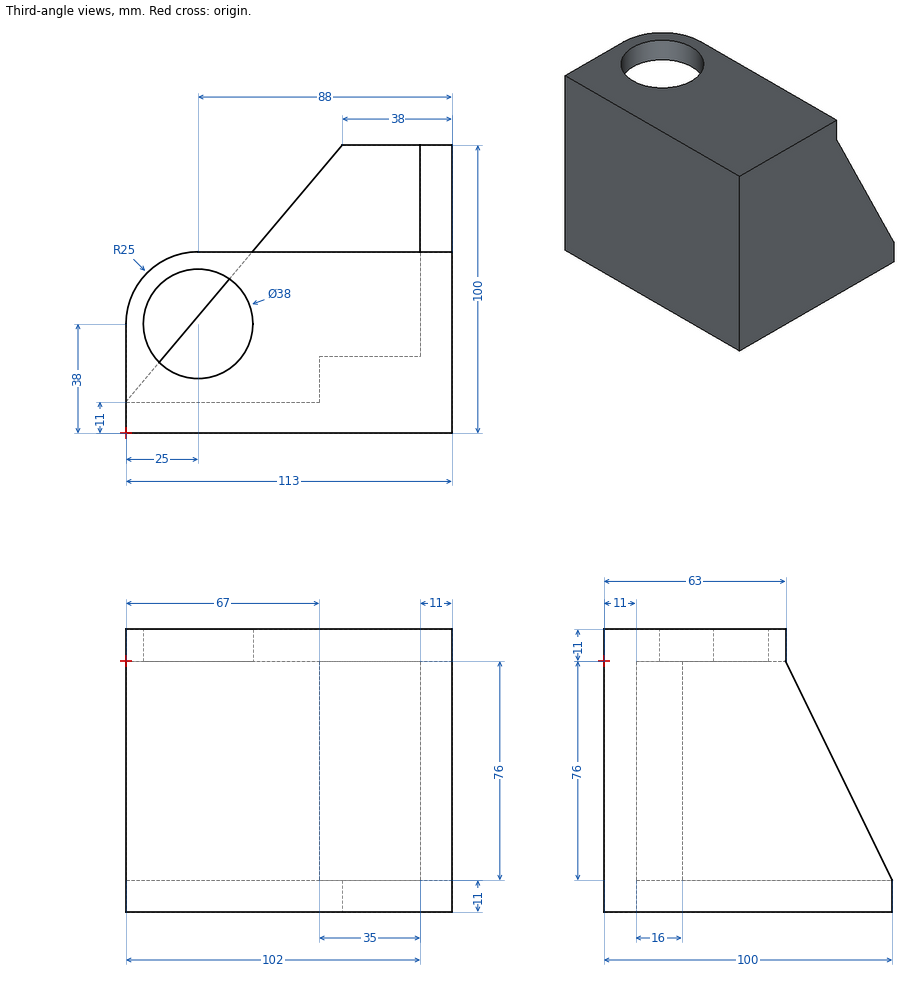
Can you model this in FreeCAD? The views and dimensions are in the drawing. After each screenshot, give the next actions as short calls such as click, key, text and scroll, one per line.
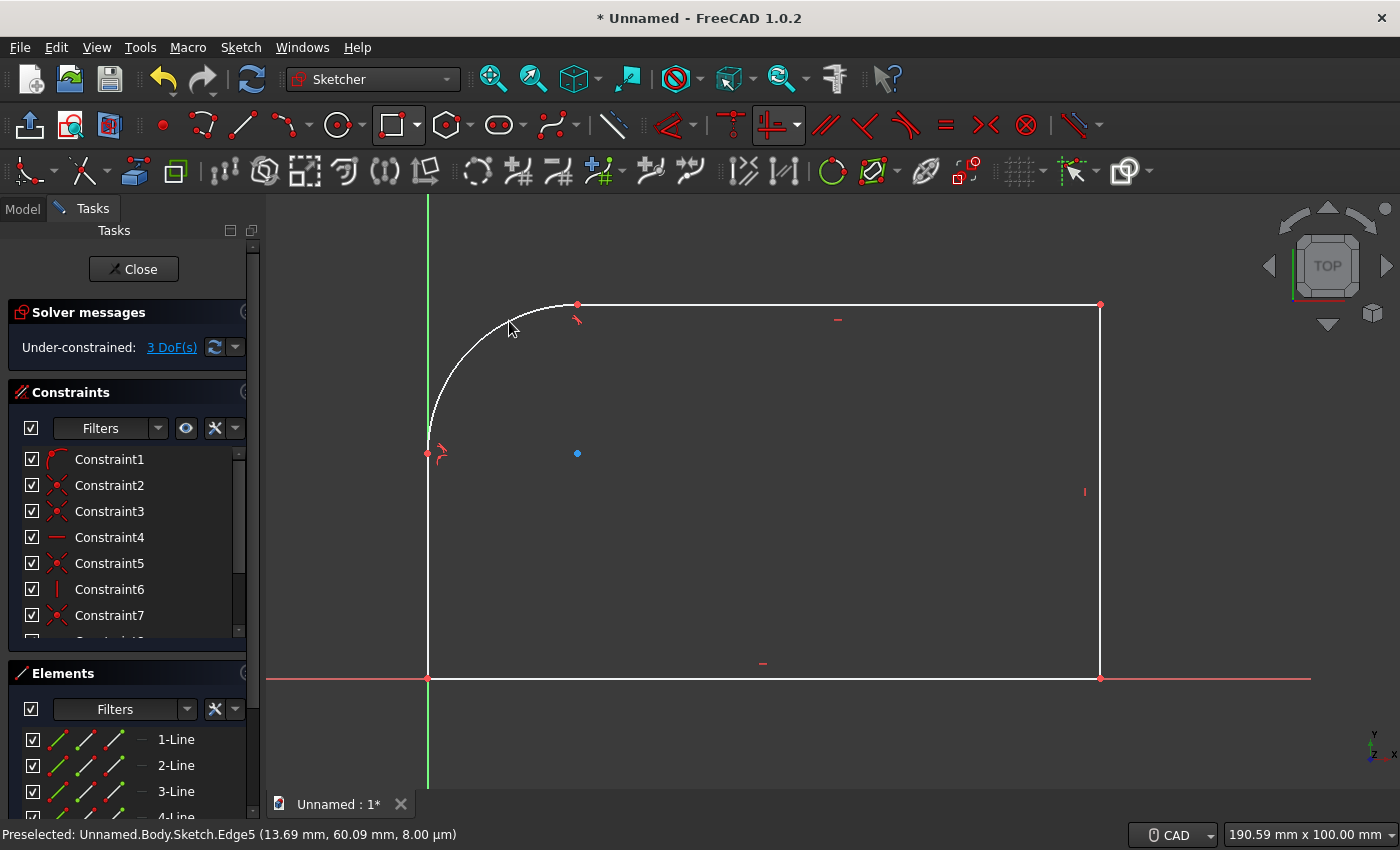
click(668, 126)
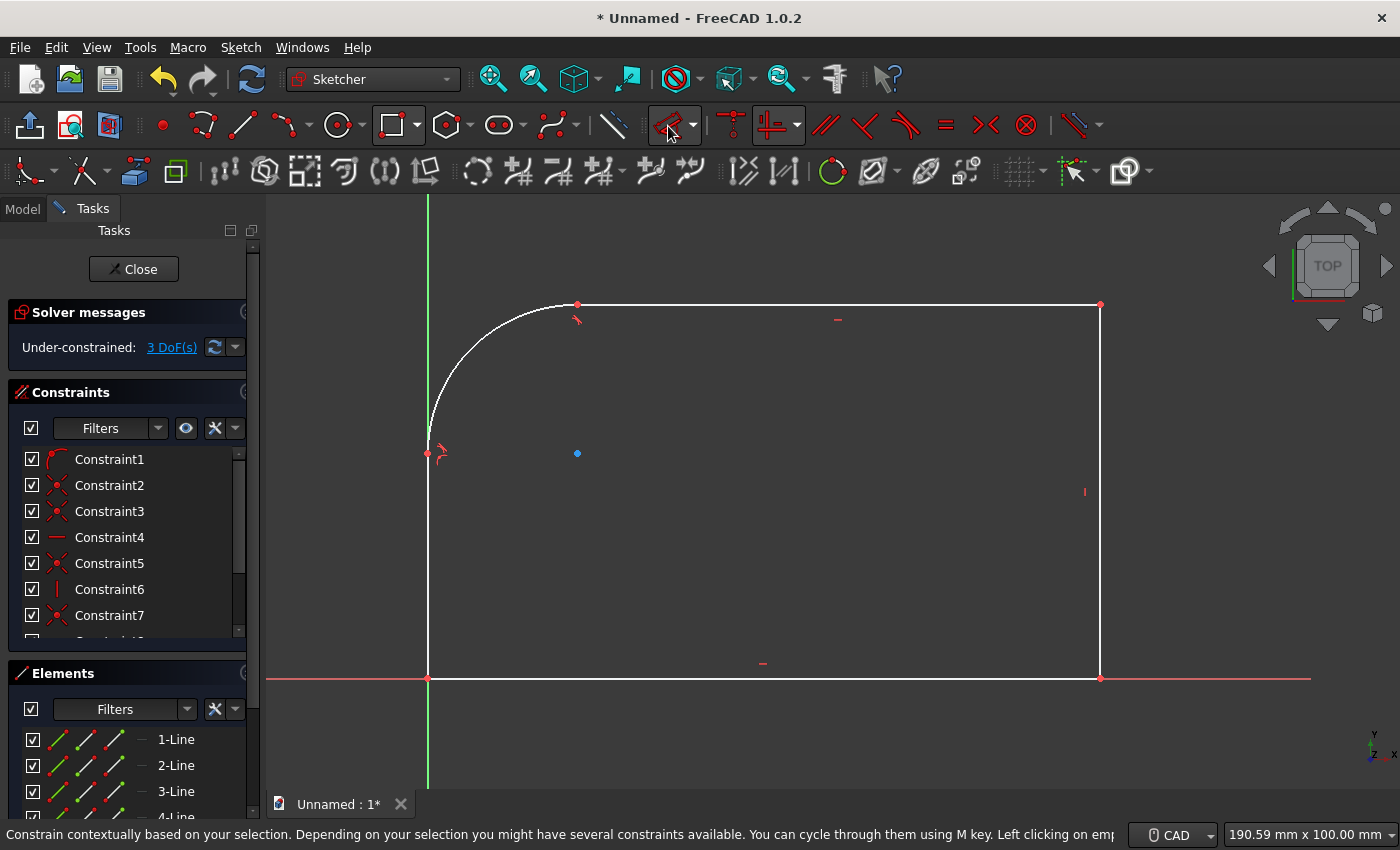
click(509, 321)
click(494, 293)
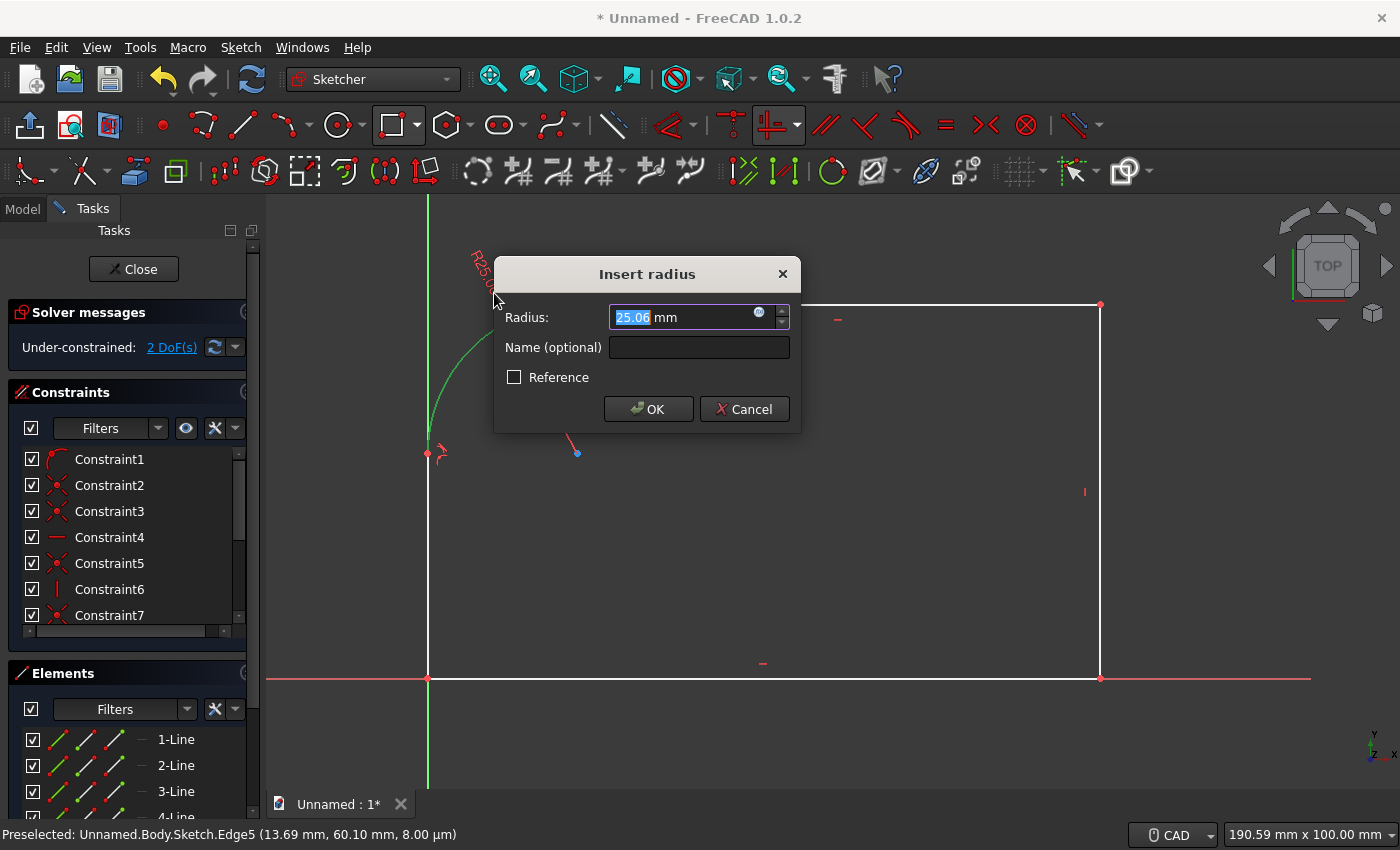
text(25)
key(Return)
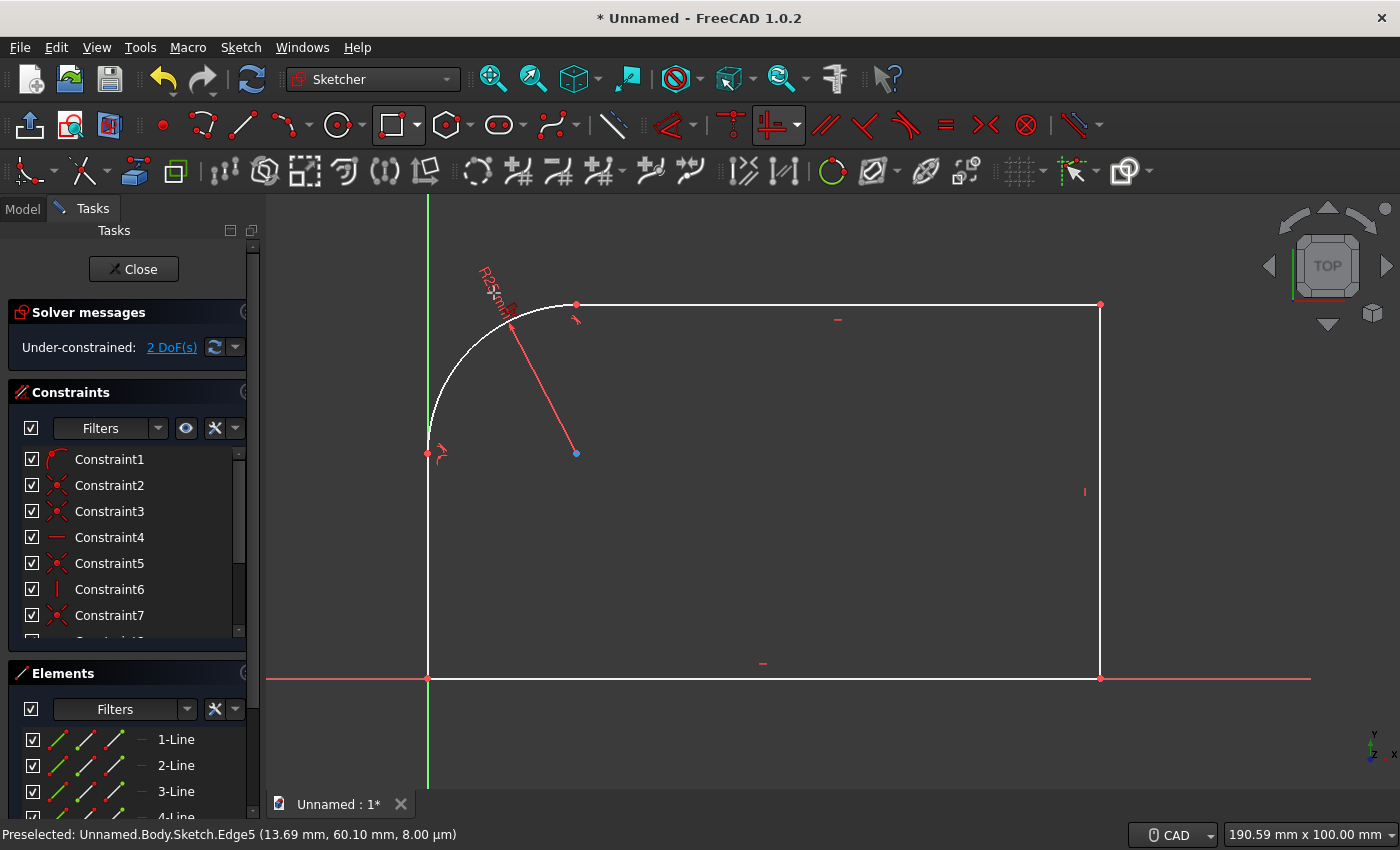
click(428, 521)
click(394, 566)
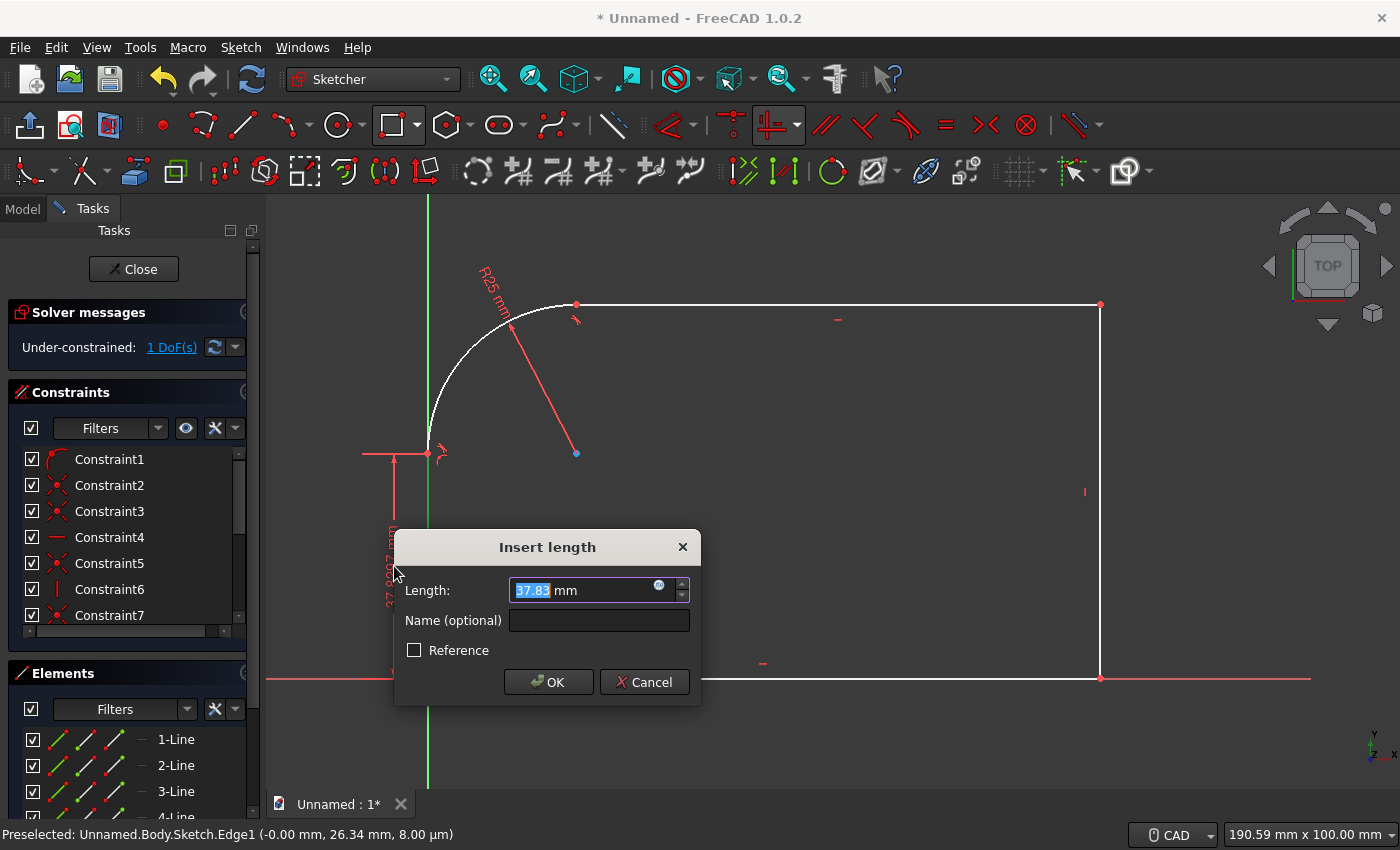
text(38)
key(Return)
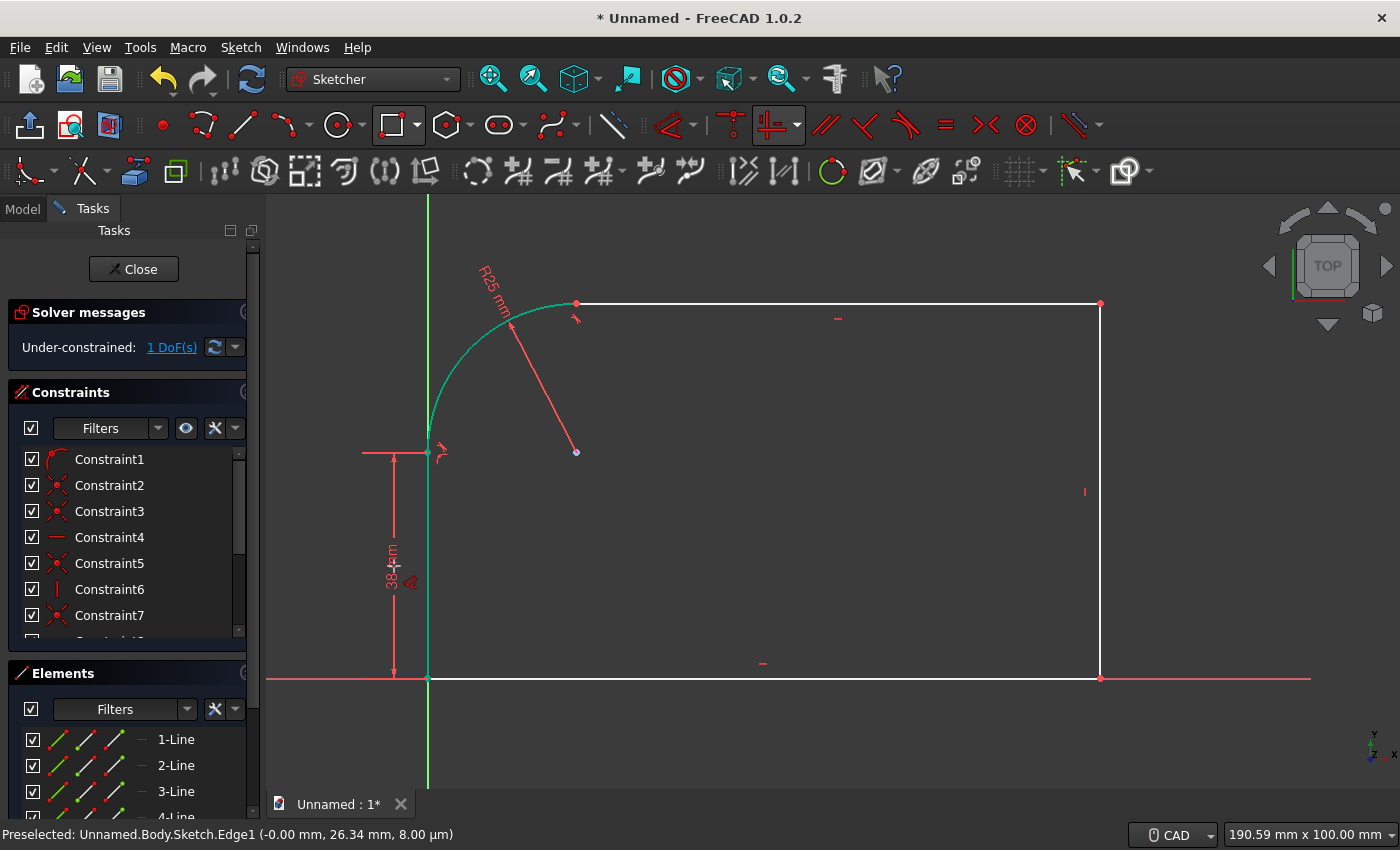
click(943, 304)
click(838, 270)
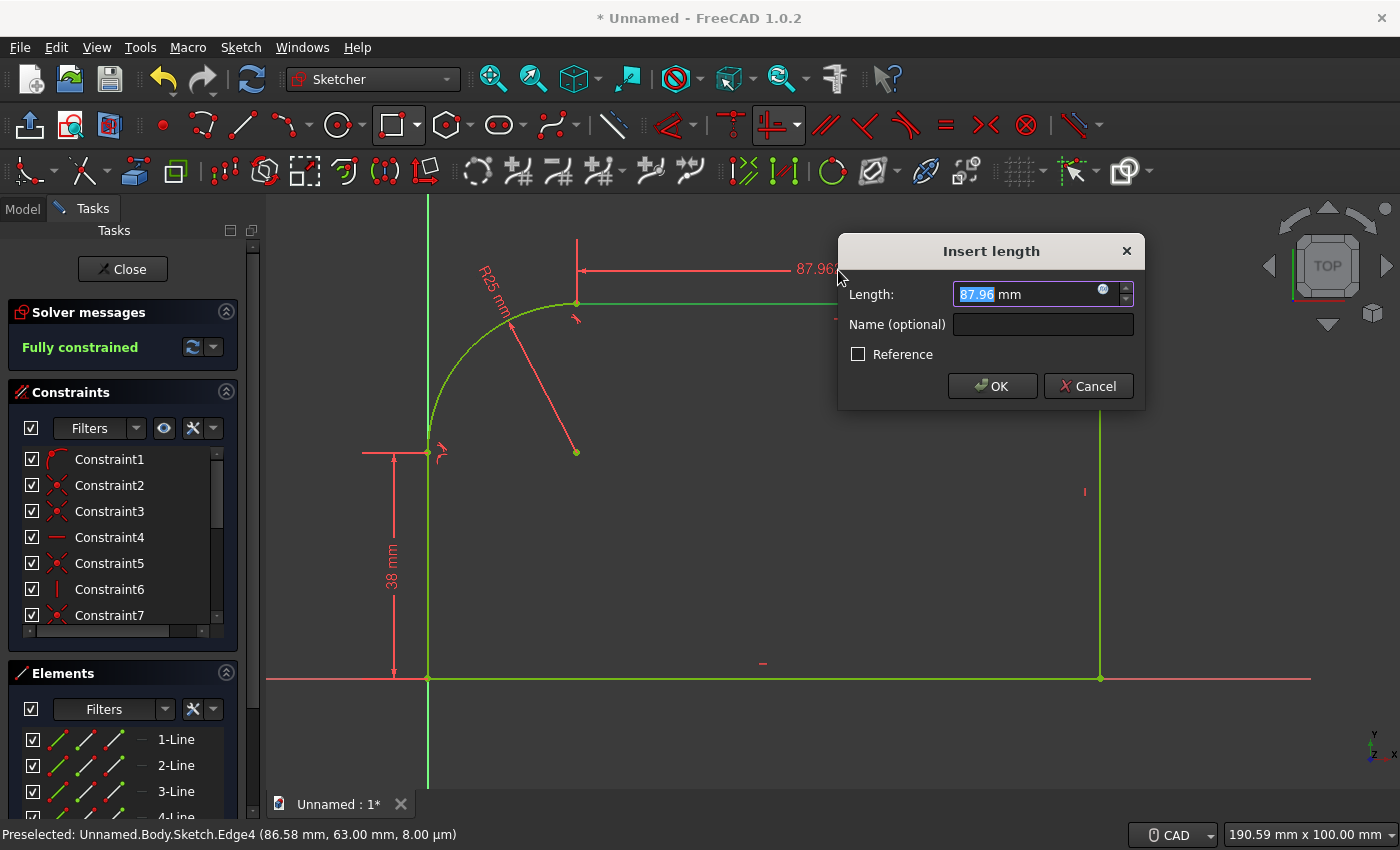
text(88)
key(Return)
key(Escape)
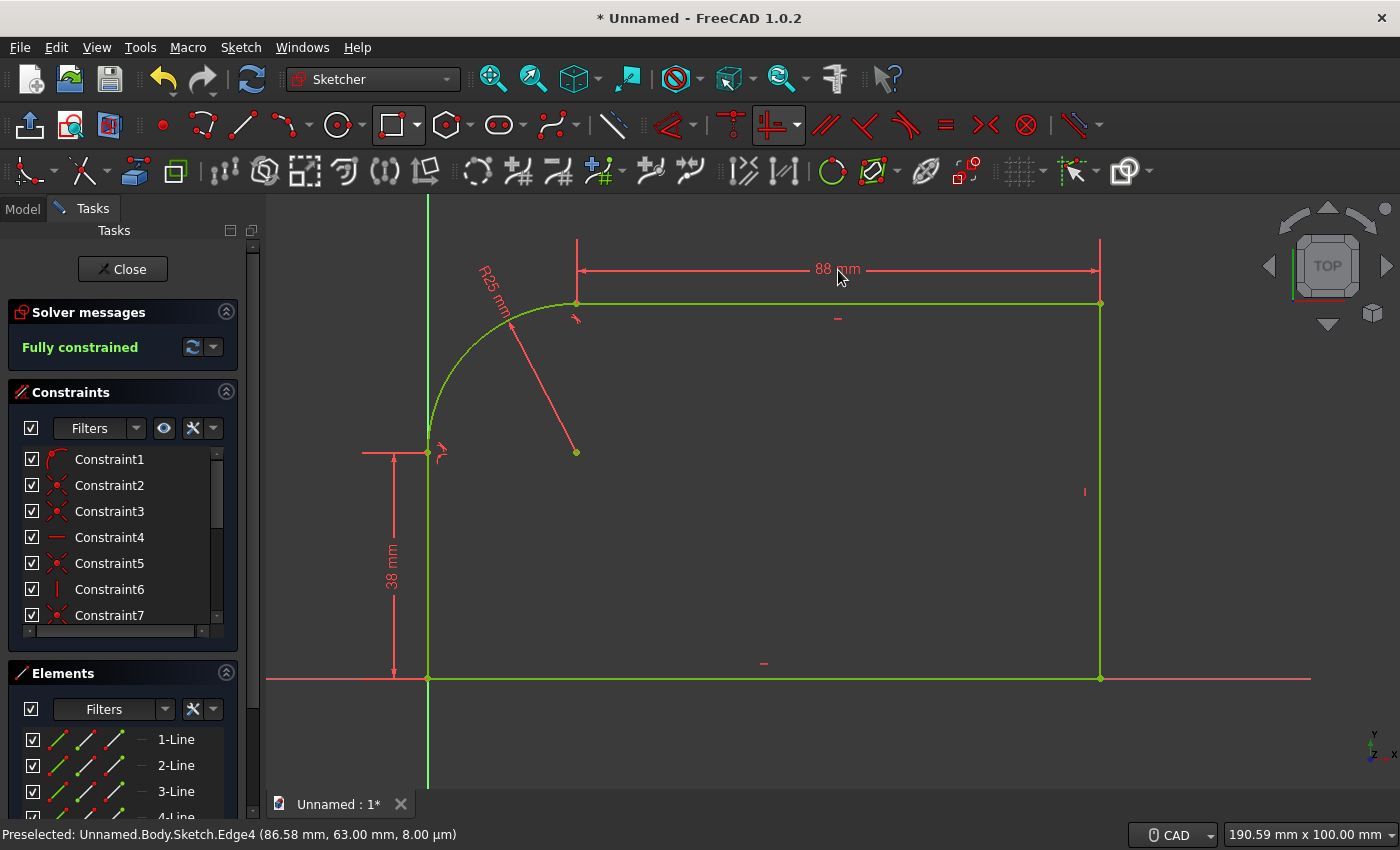
click(123, 269)